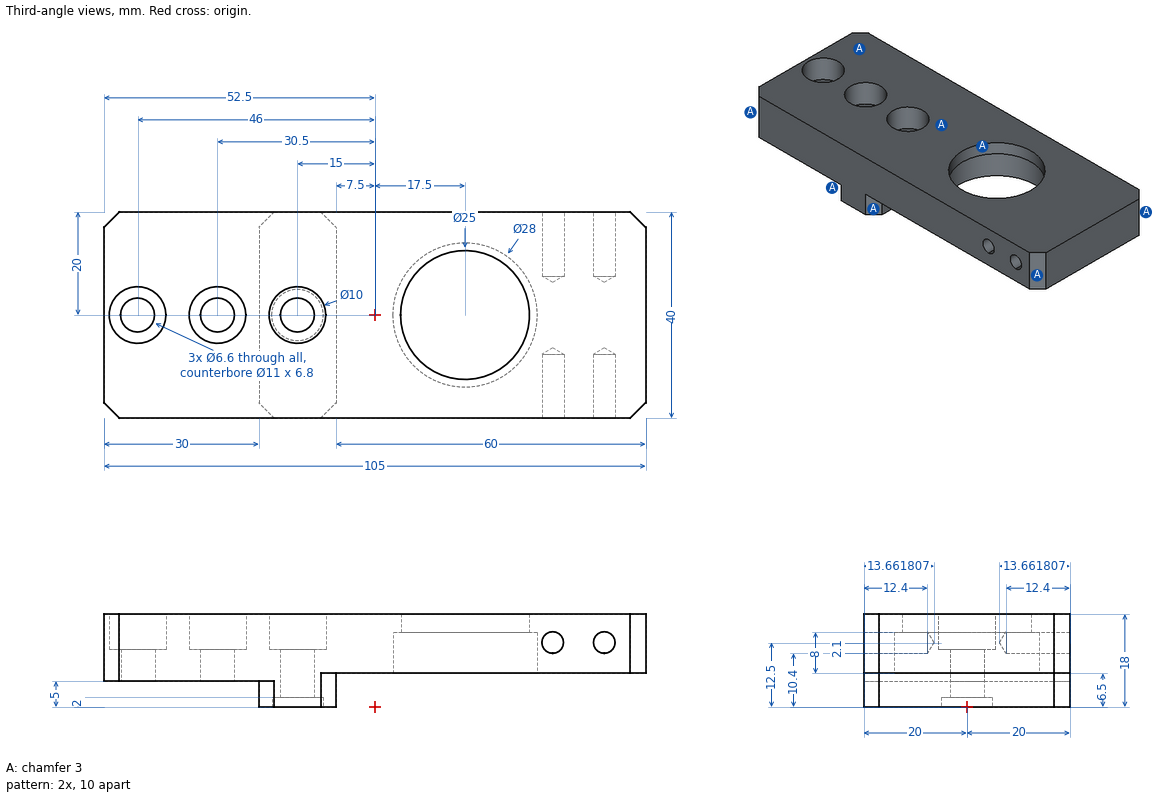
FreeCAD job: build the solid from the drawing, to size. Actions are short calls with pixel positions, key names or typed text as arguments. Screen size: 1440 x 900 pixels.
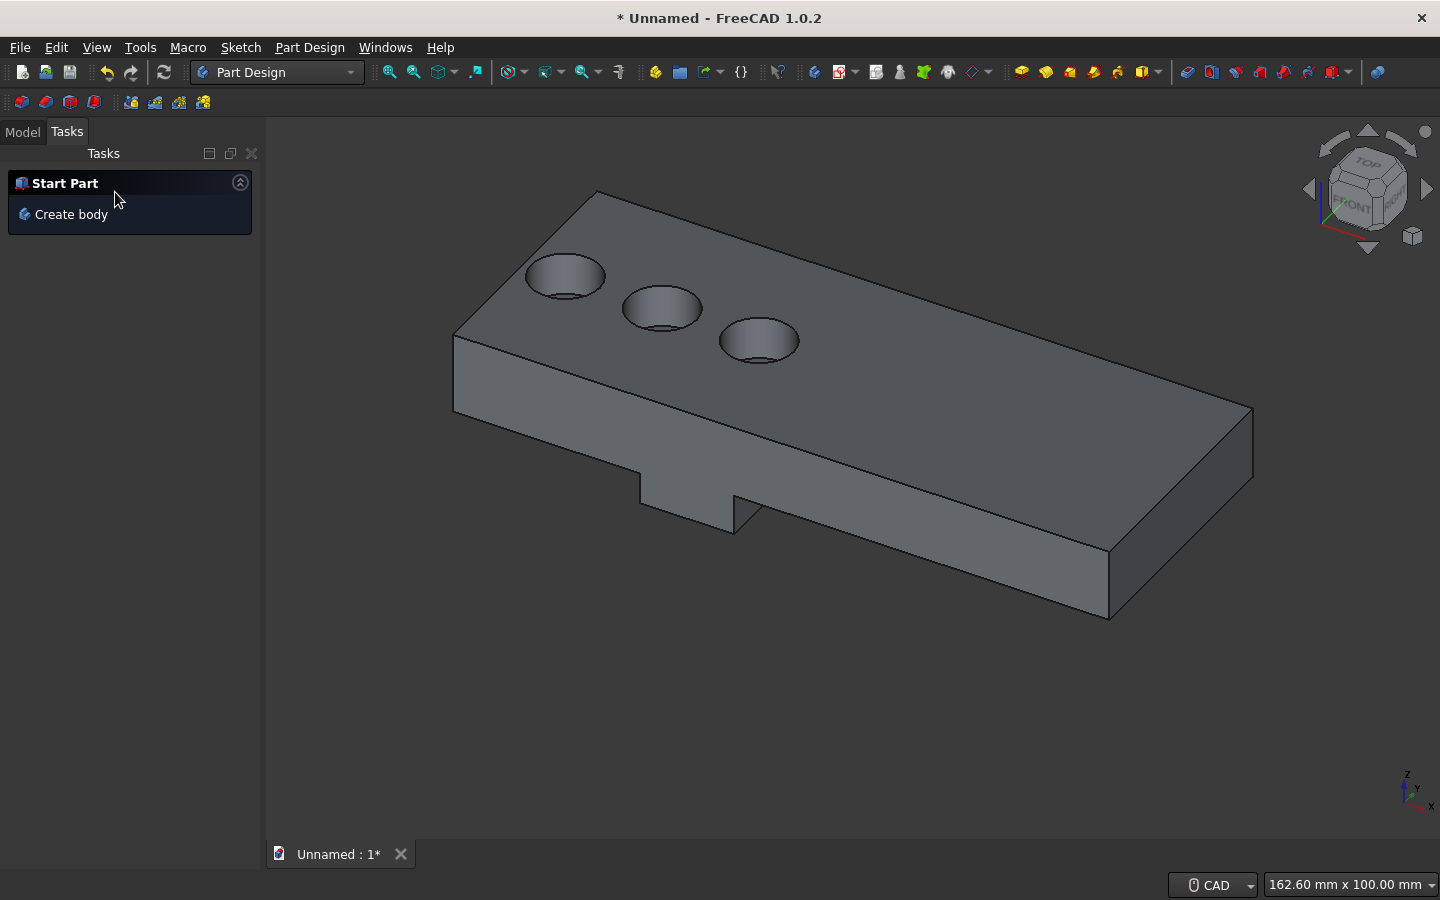
key(5)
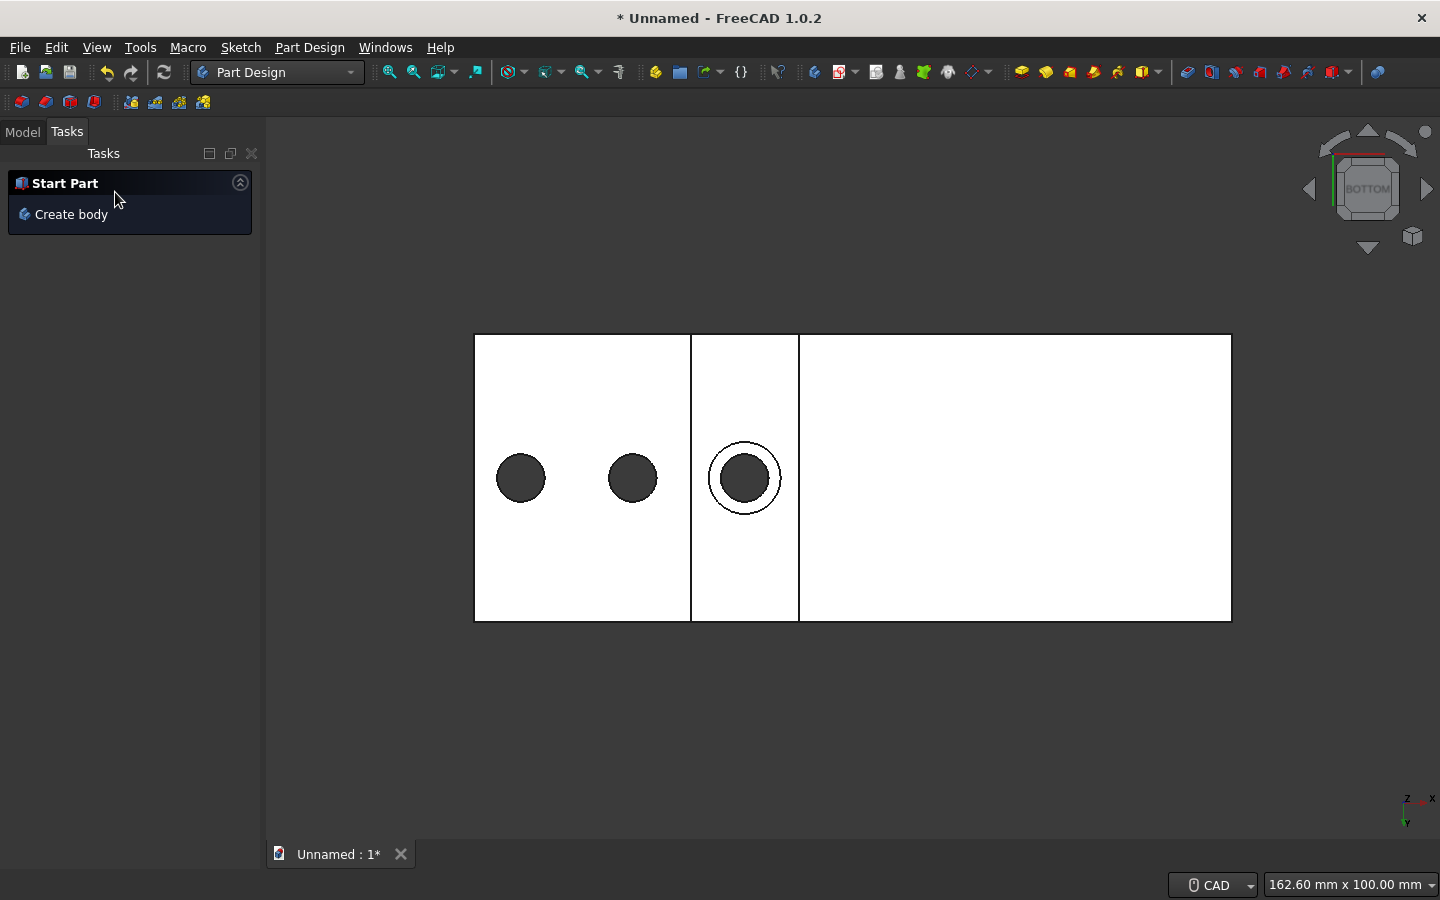
click(1077, 477)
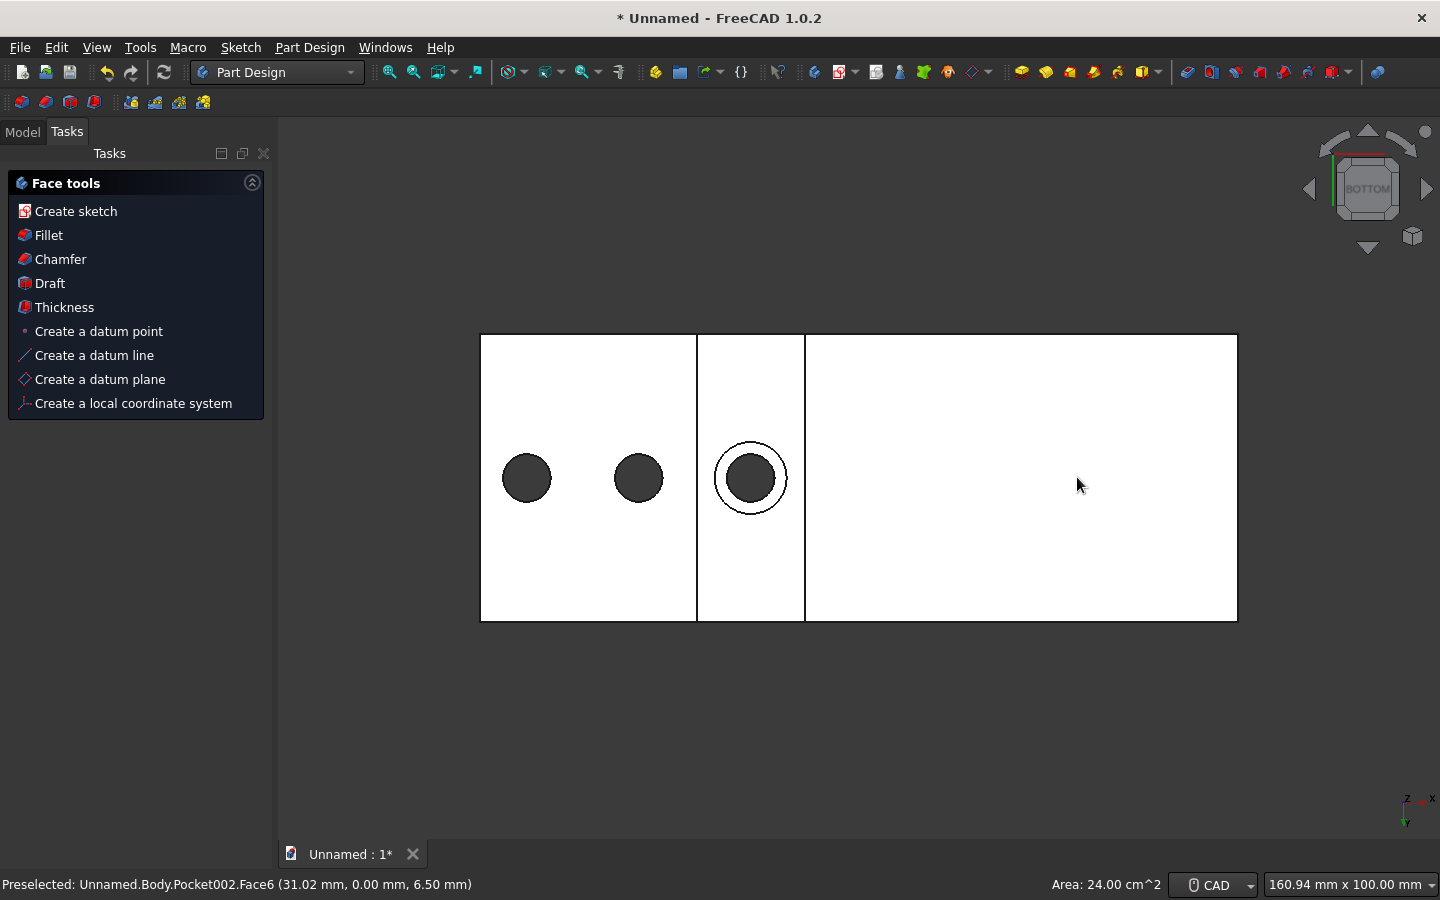
click(840, 72)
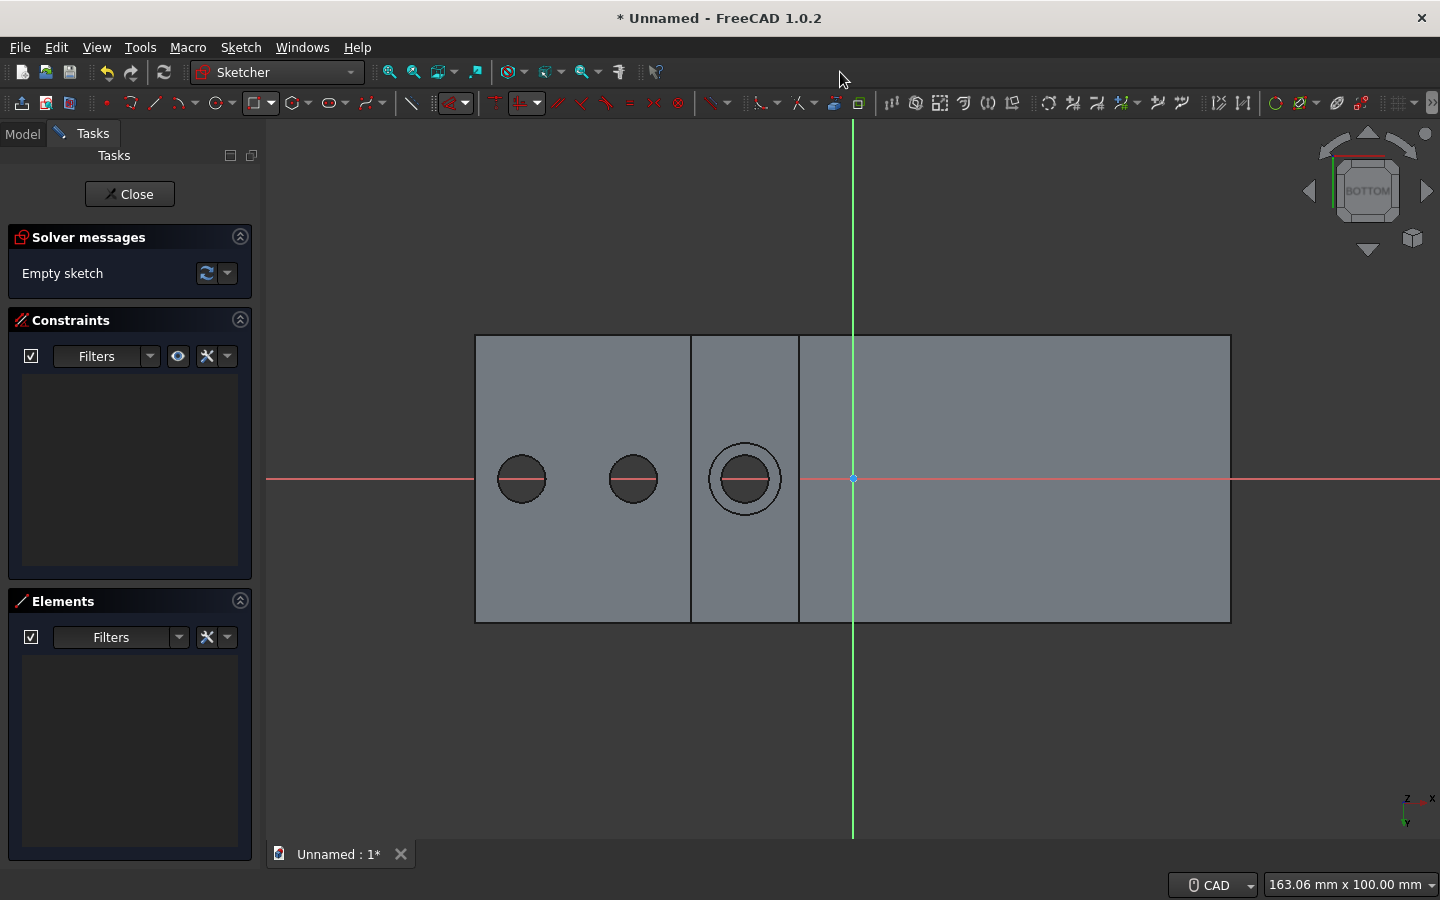
scroll(1115, 479, up, 4)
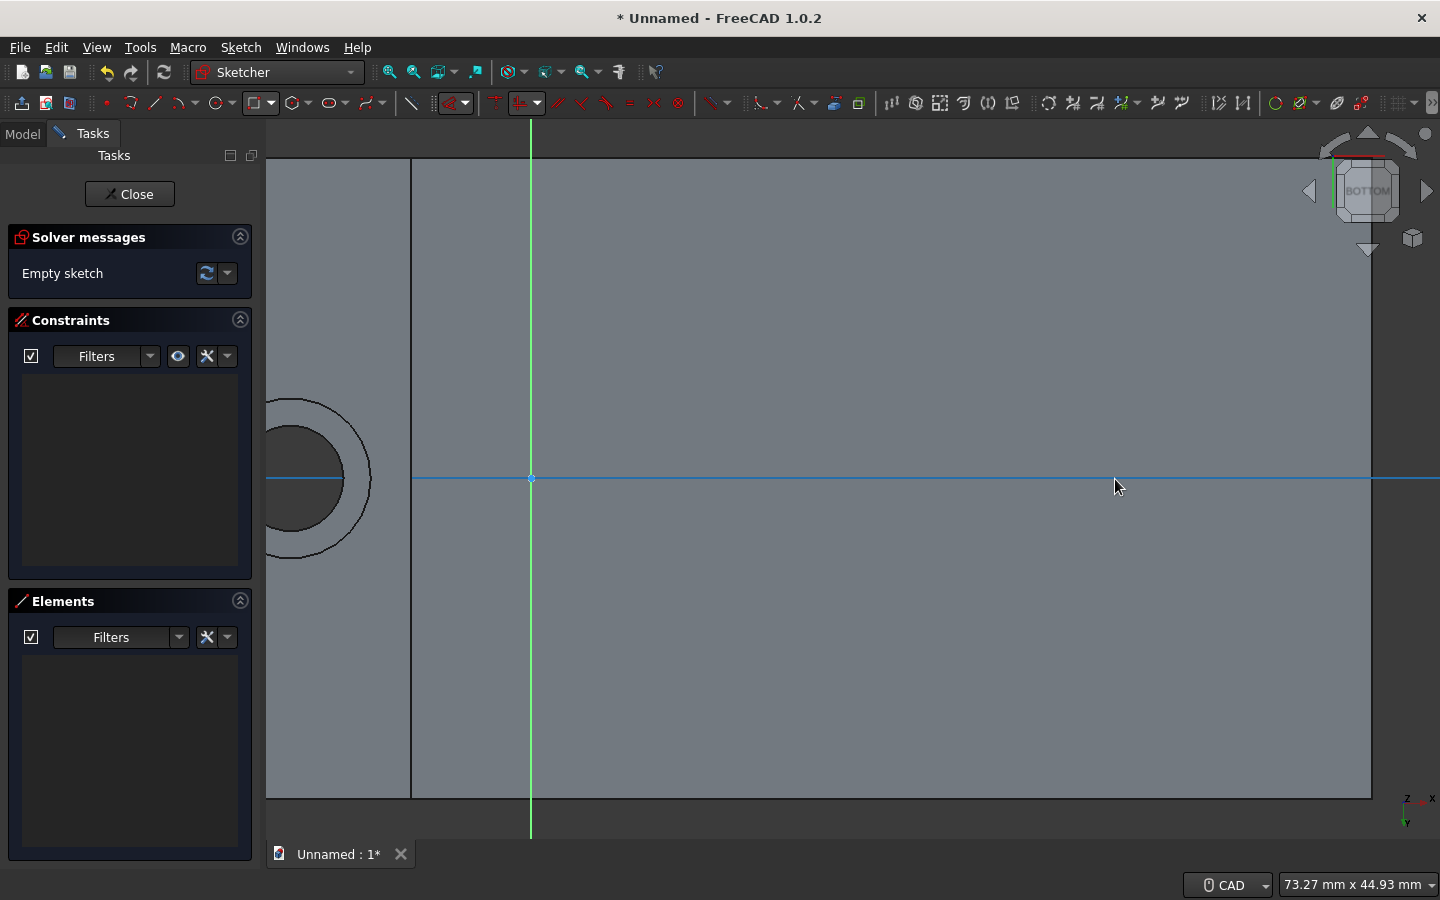
click(216, 104)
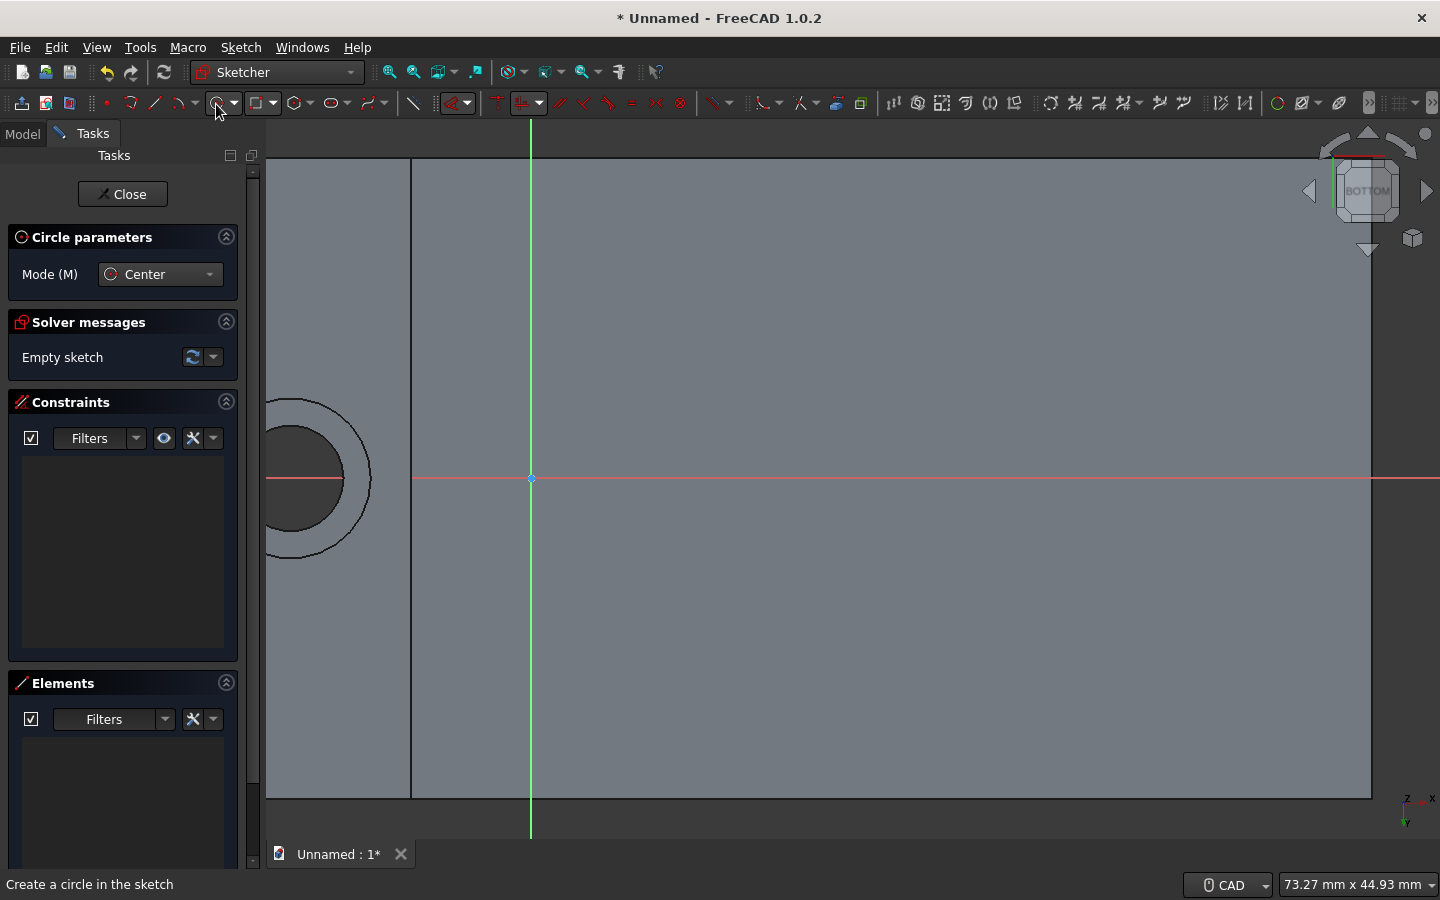
click(811, 478)
click(970, 320)
key(Escape)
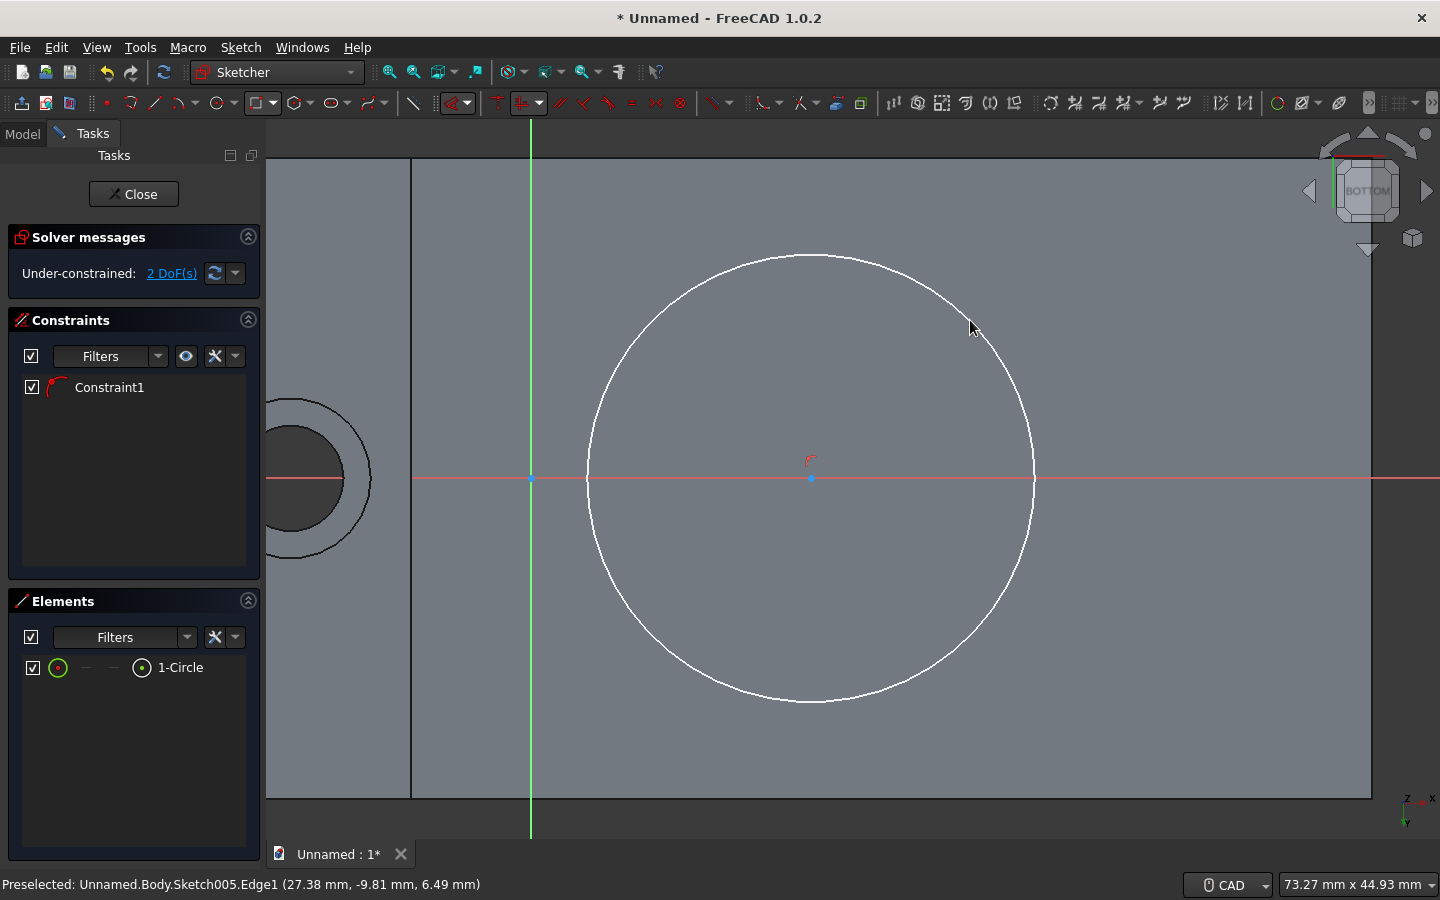
click(969, 320)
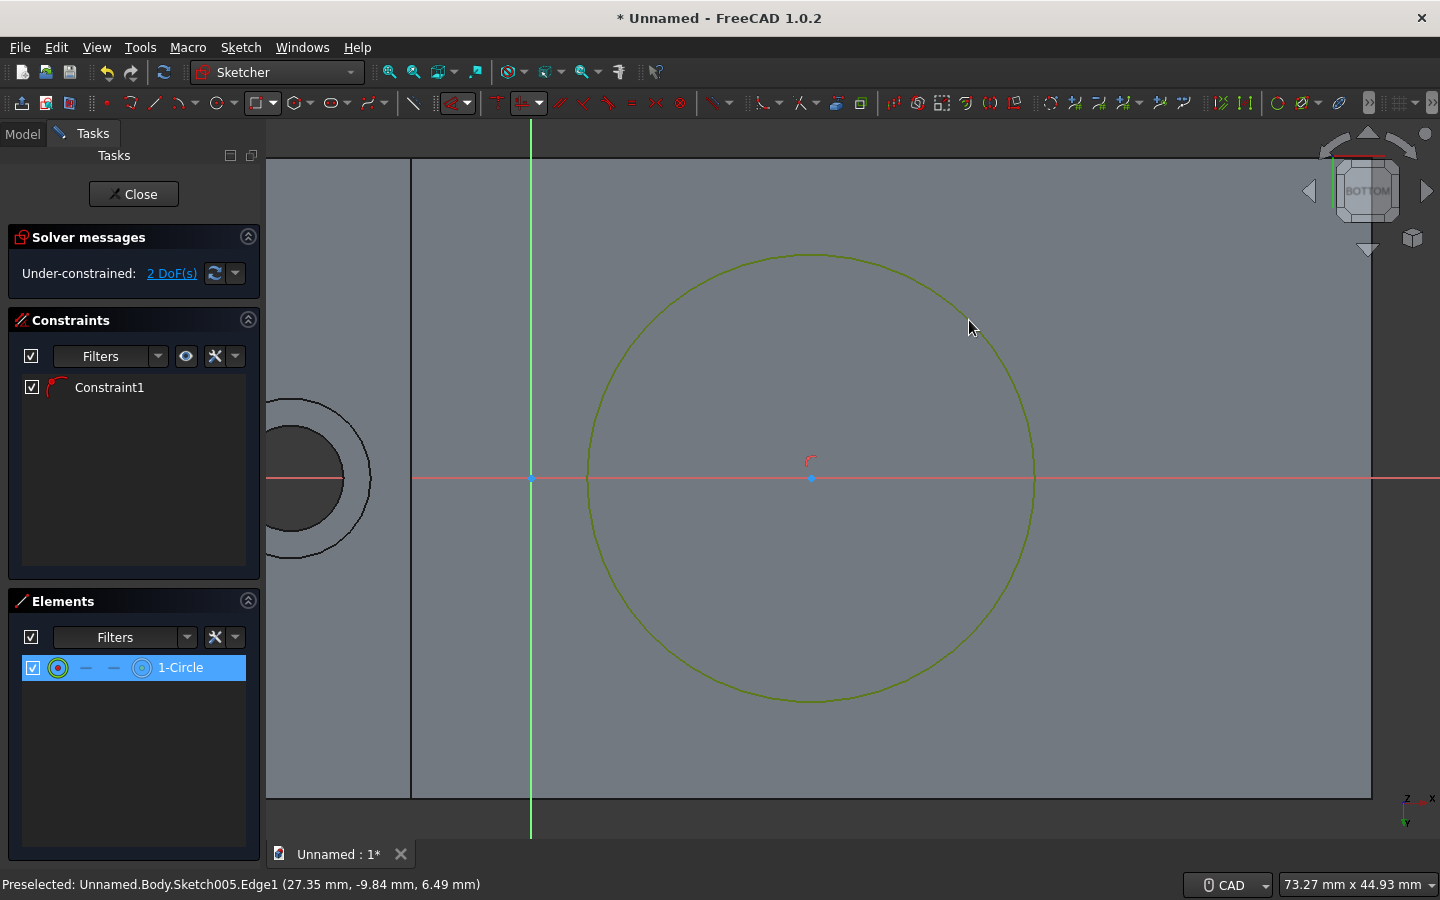
click(470, 104)